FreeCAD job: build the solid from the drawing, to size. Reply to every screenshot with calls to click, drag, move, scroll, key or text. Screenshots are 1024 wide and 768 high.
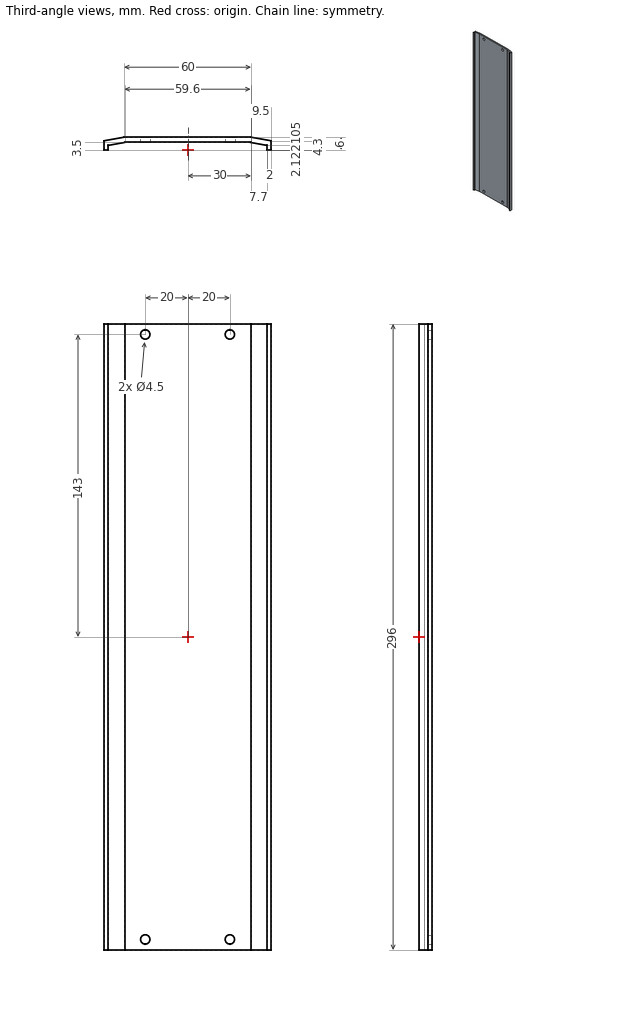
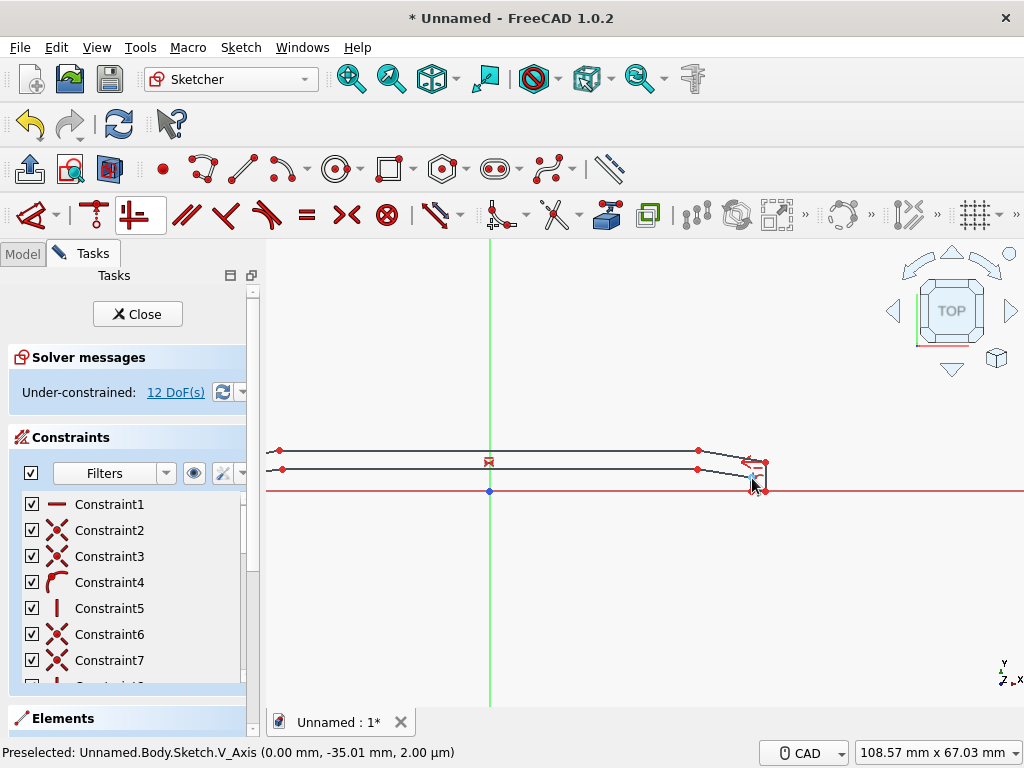
click(751, 478)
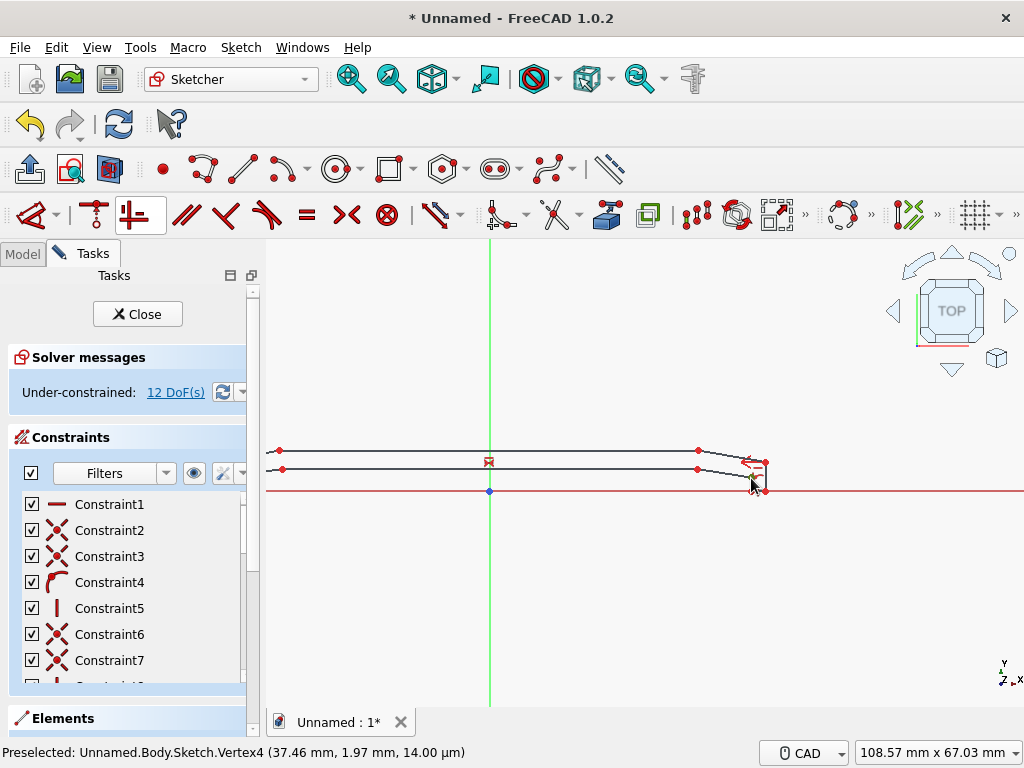
scroll(753, 478, down, 2)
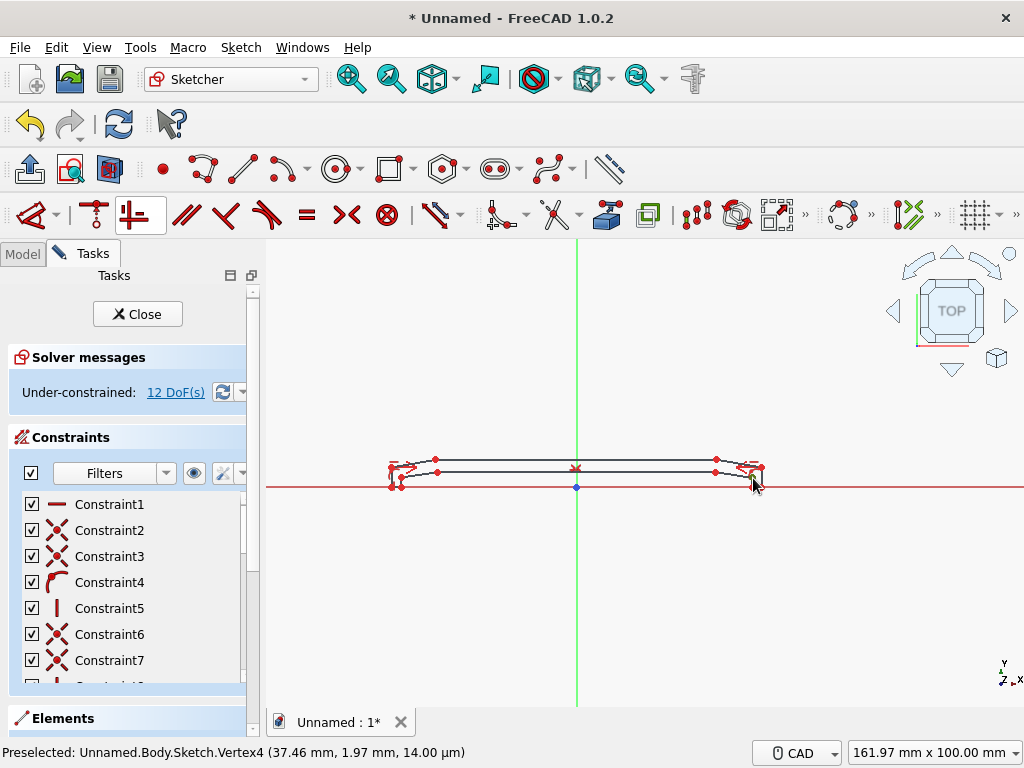
scroll(401, 478, up, 2)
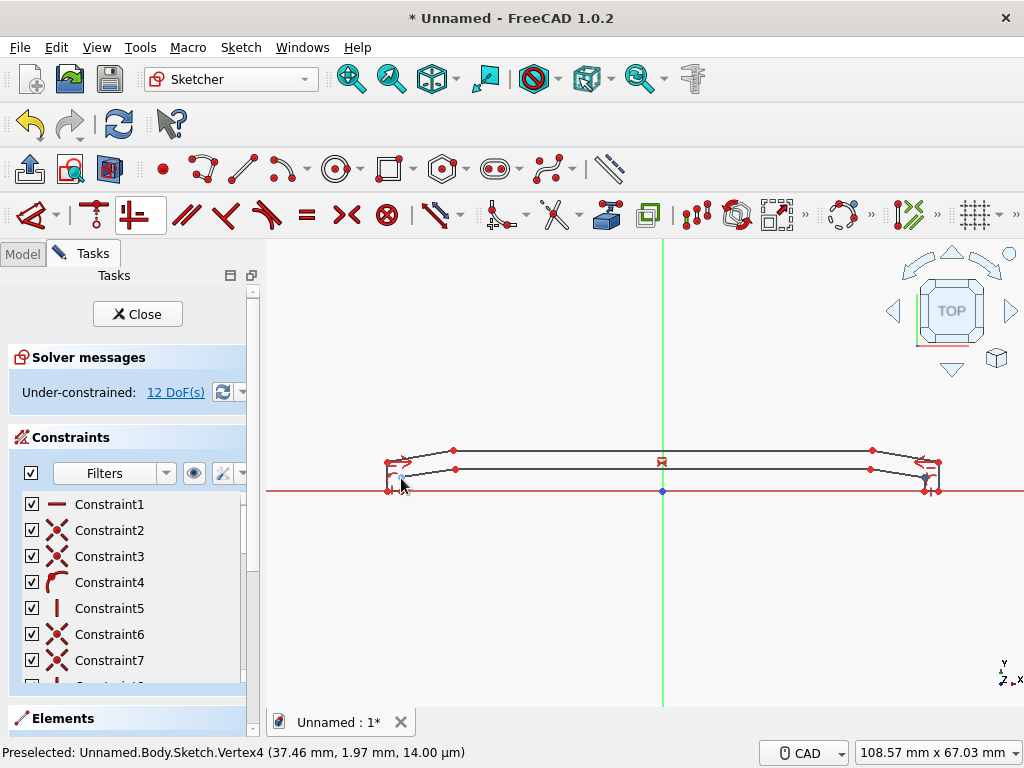
click(401, 477)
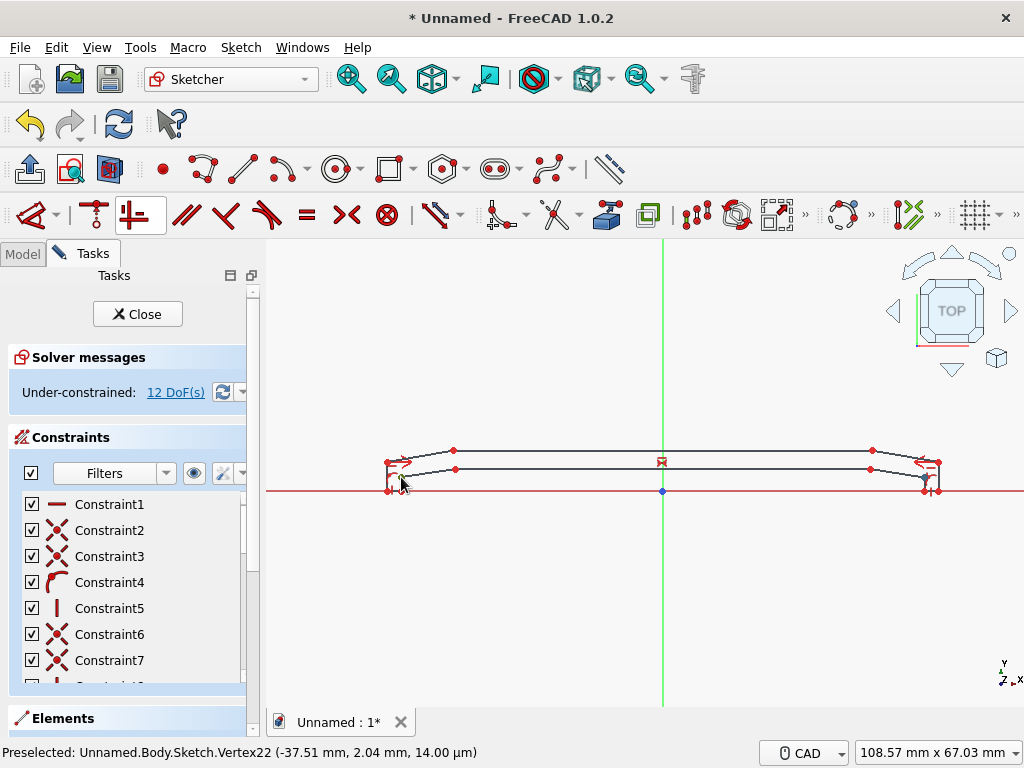
click(663, 650)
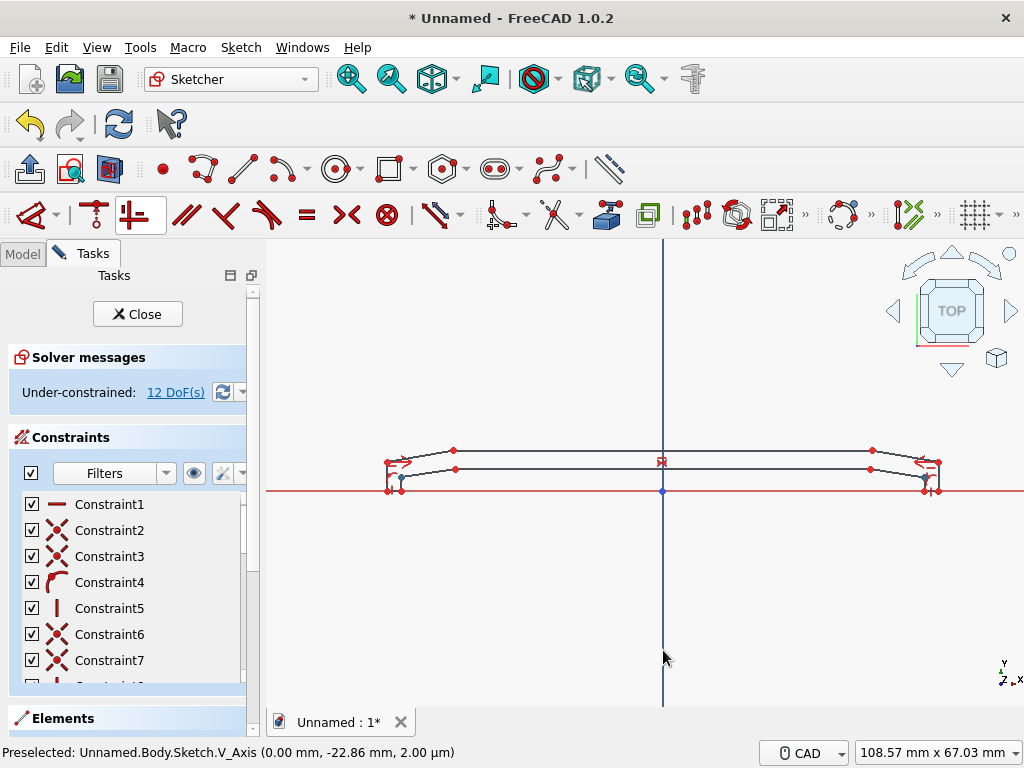
key(s)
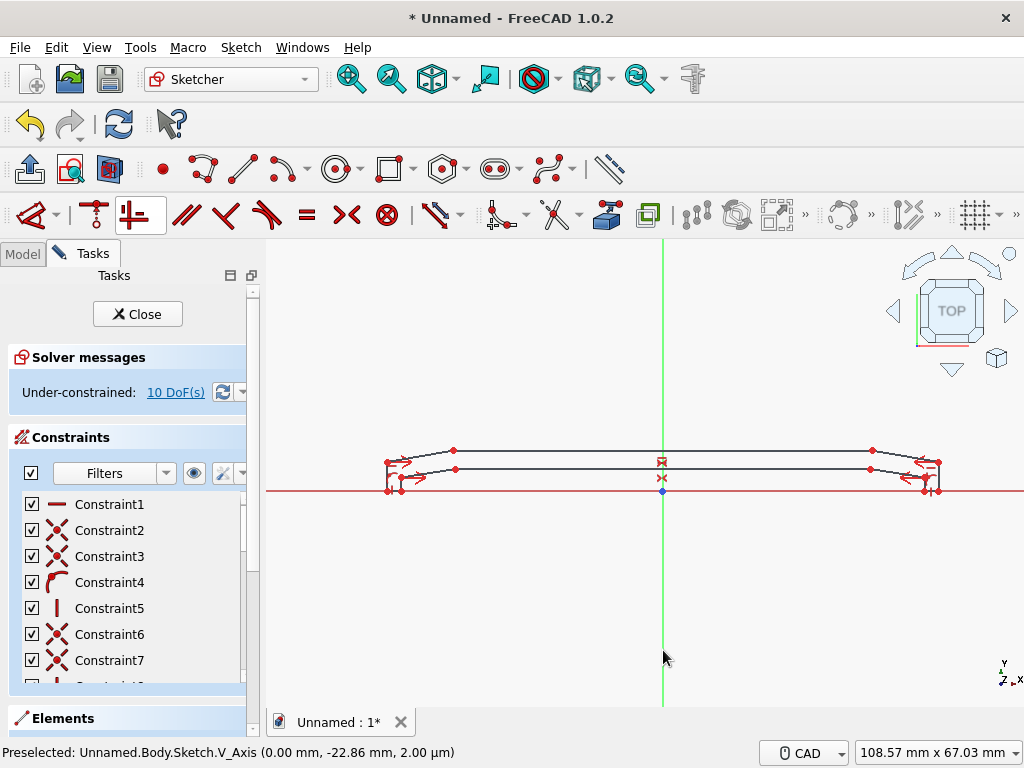
key(d)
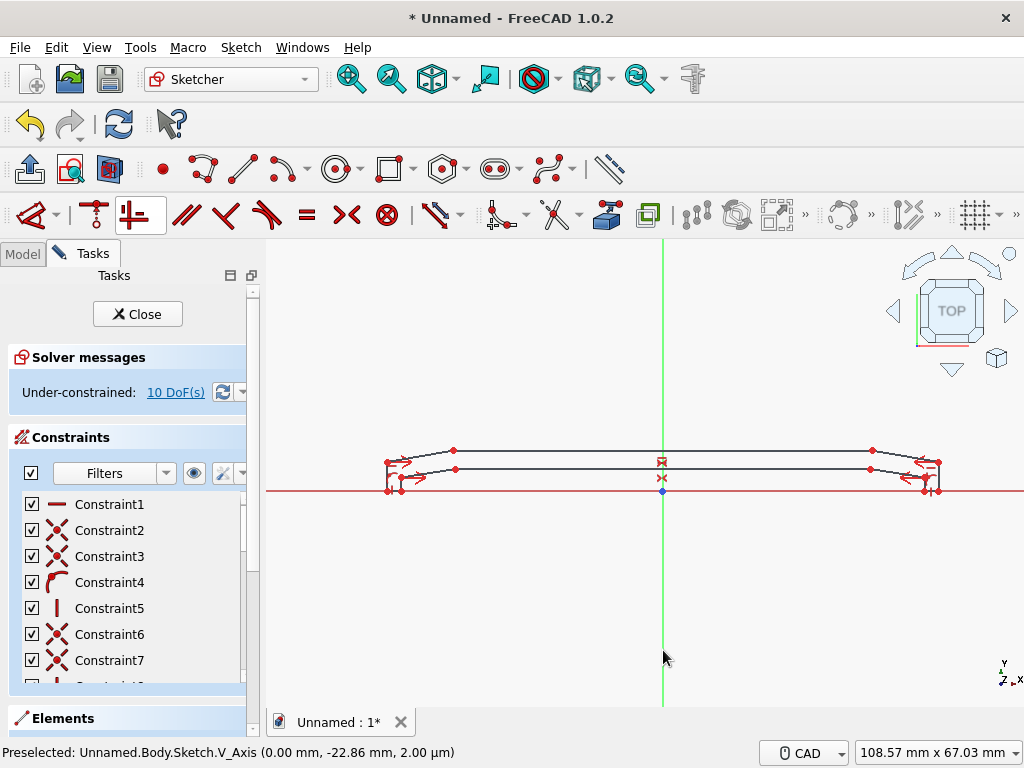
scroll(401, 478, down, 2)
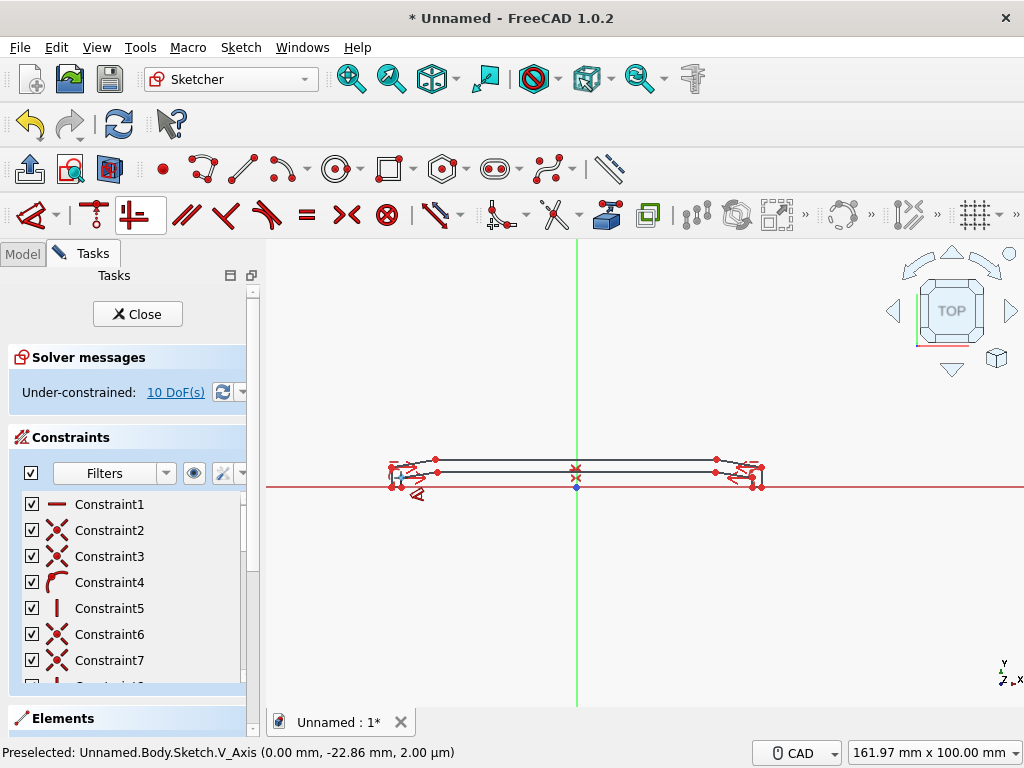
scroll(757, 487, up, 8)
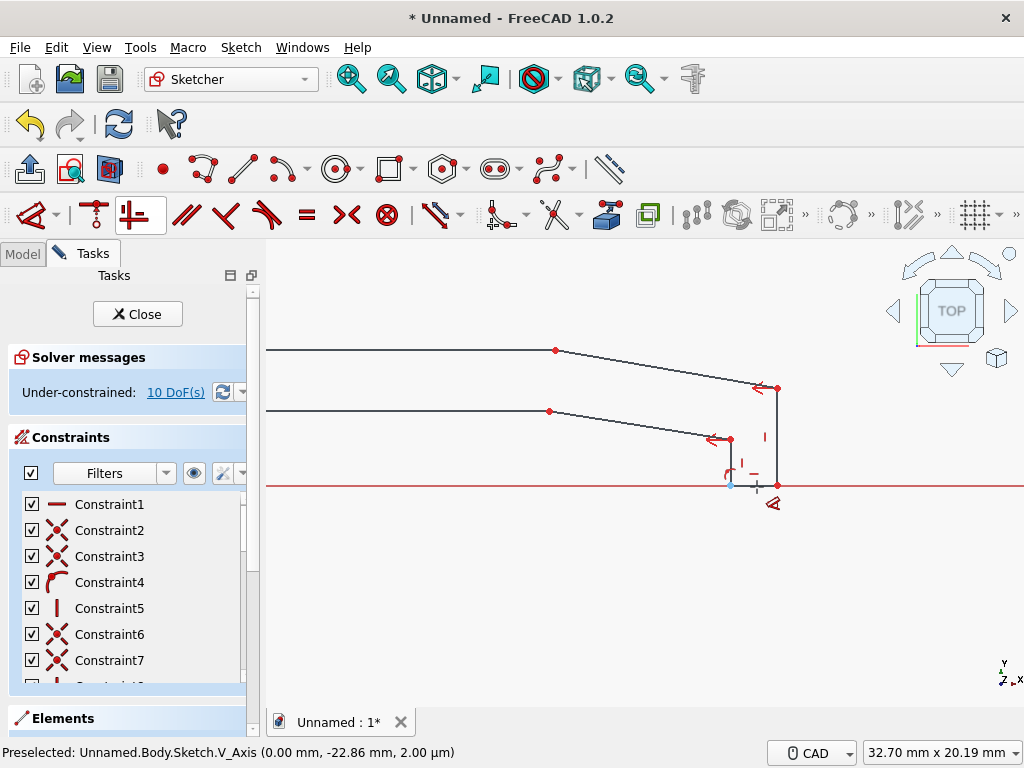
click(754, 486)
click(754, 520)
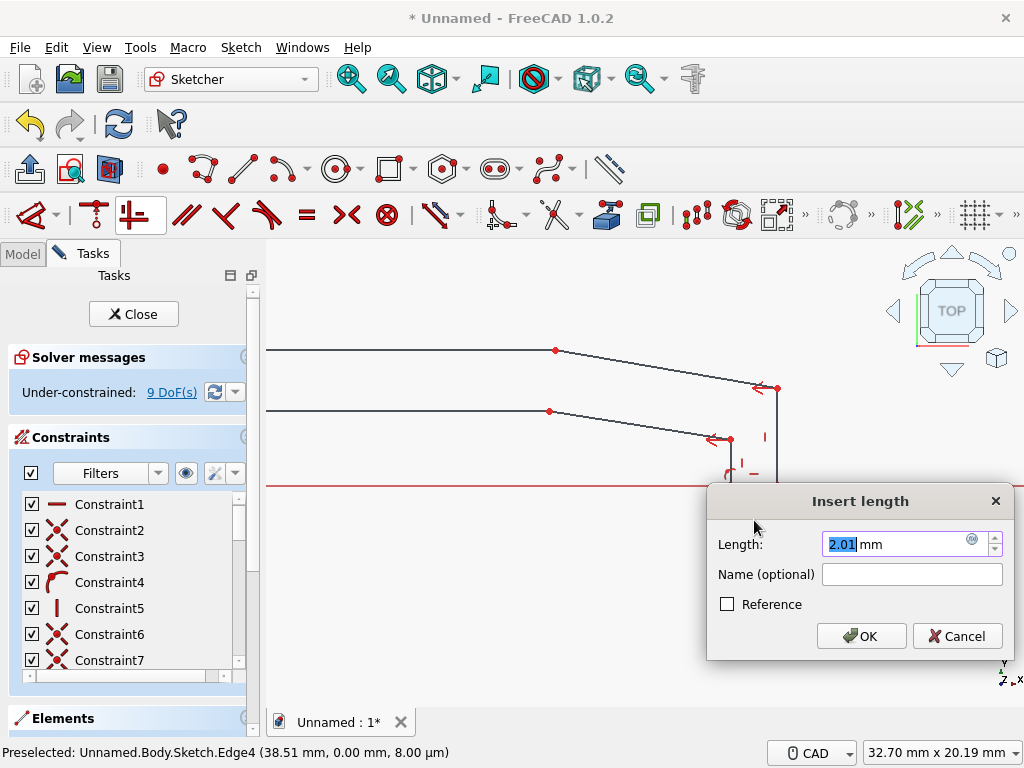
text(2)
key(Return)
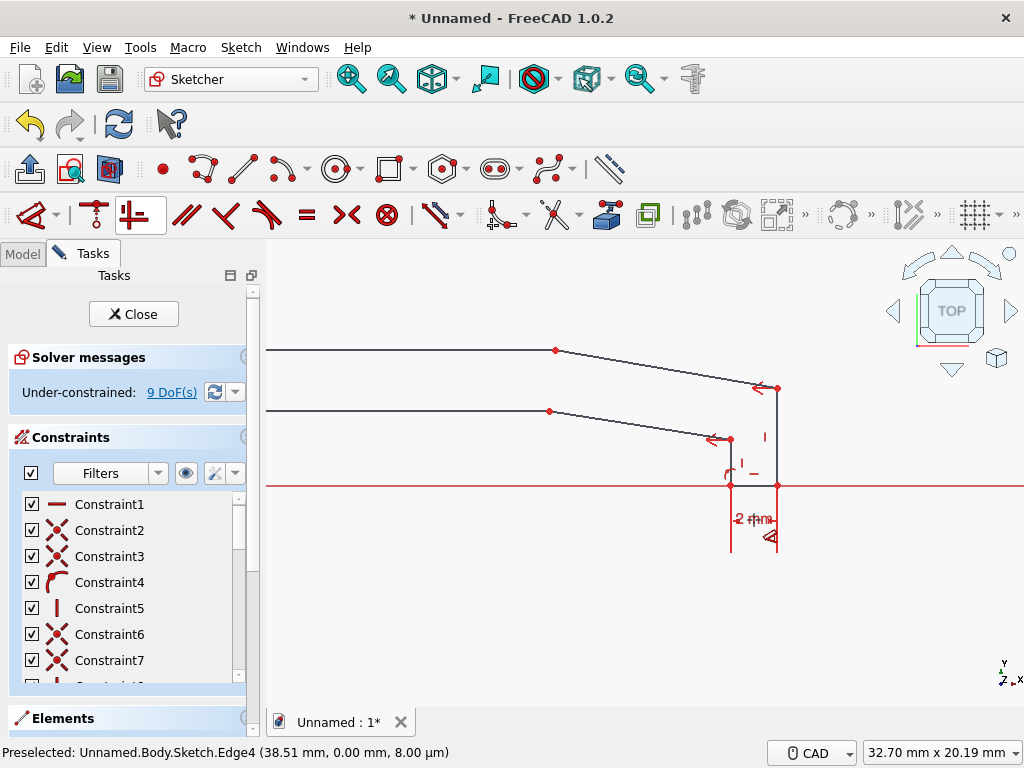
scroll(757, 487, down, 8)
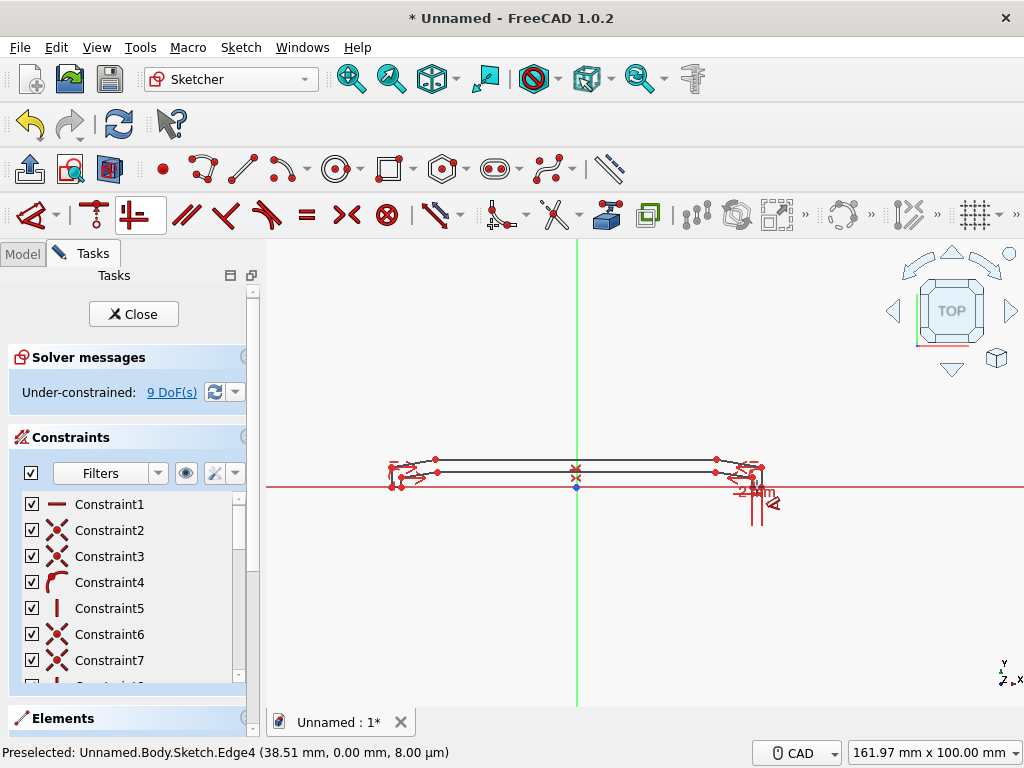
click(633, 460)
click(512, 426)